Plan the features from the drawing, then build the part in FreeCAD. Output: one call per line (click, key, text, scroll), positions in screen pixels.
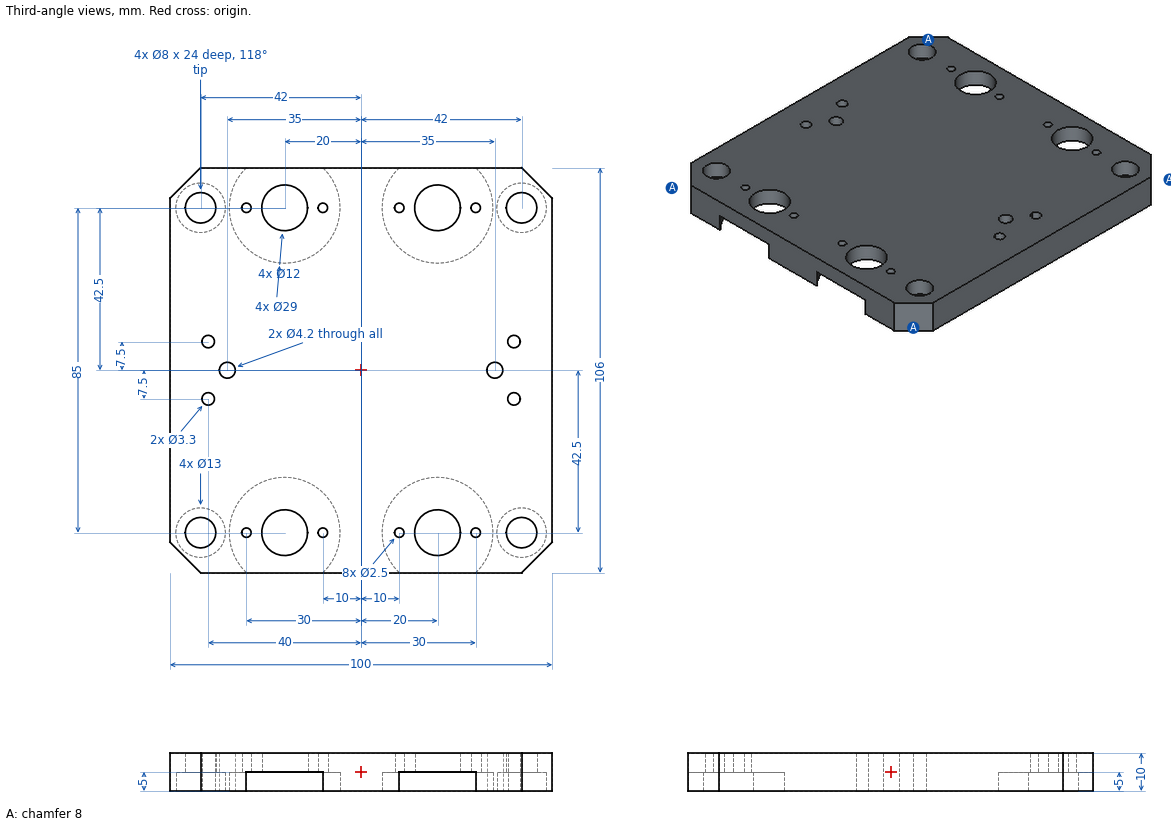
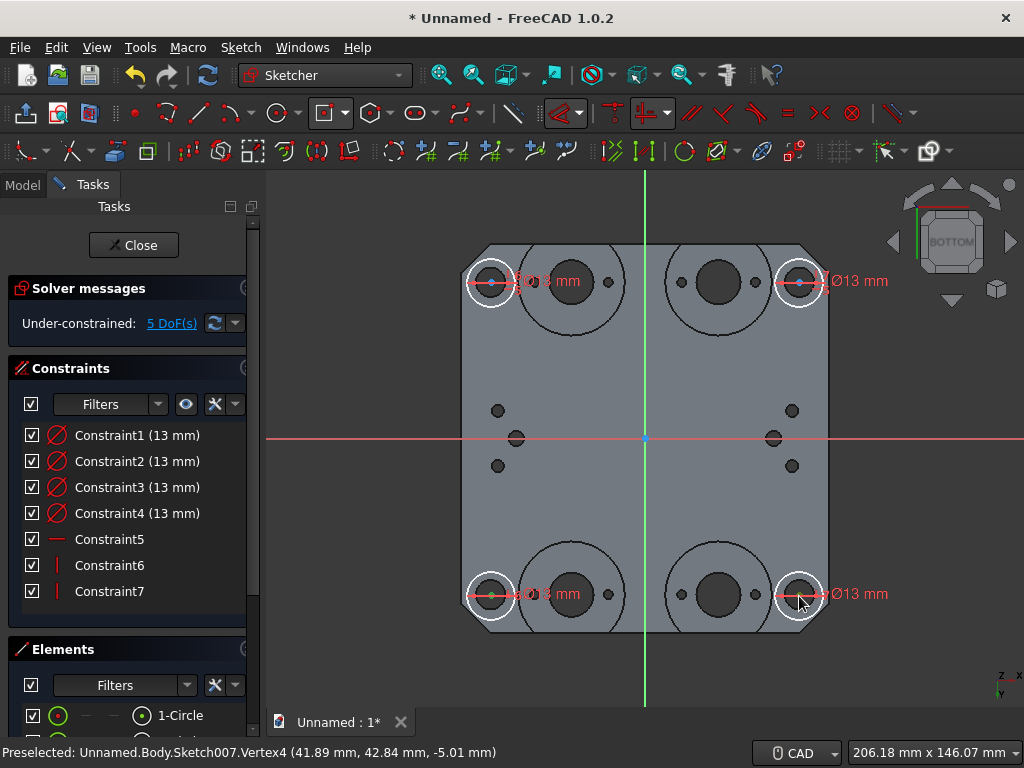
key(h)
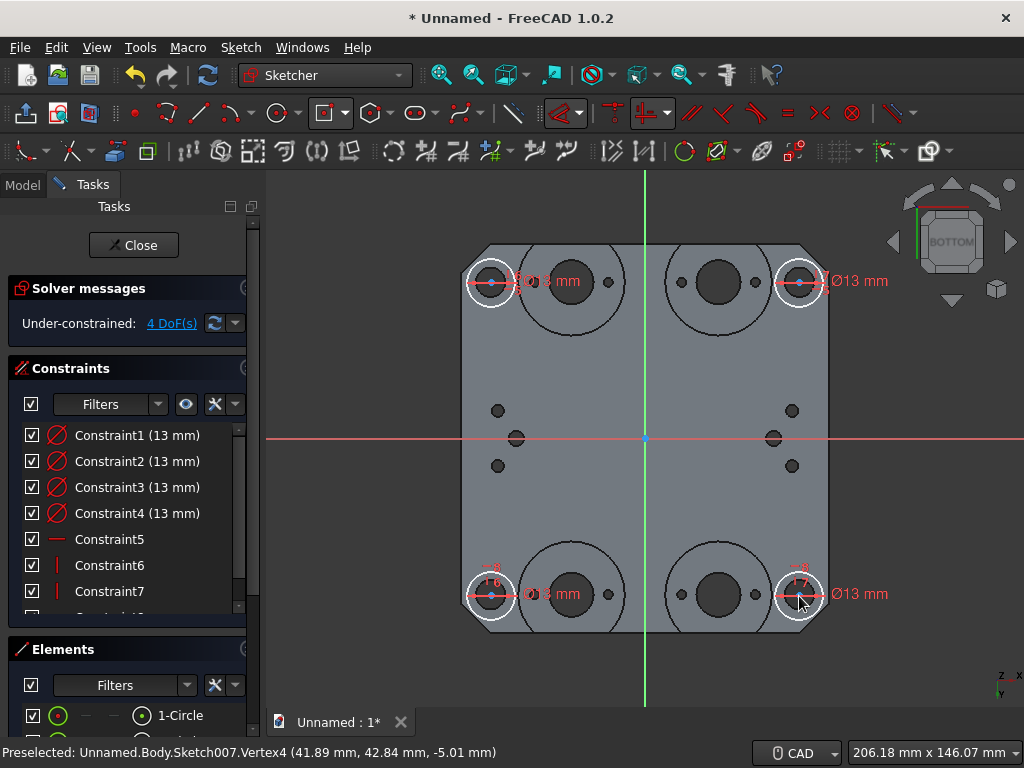
click(491, 283)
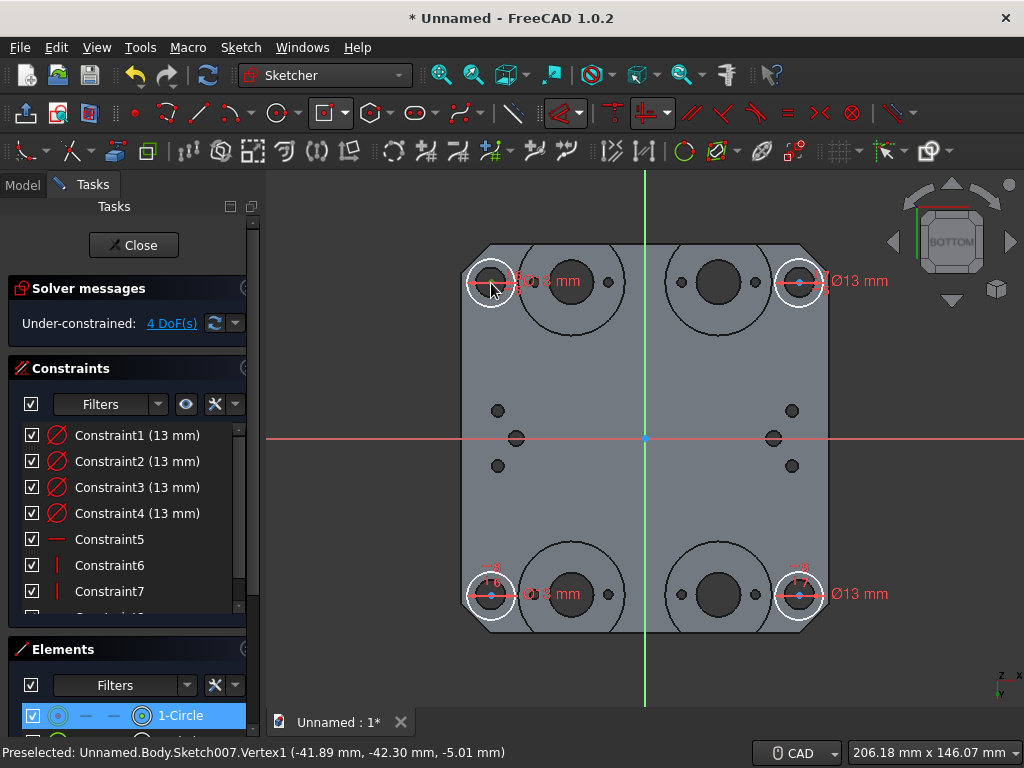
click(582, 114)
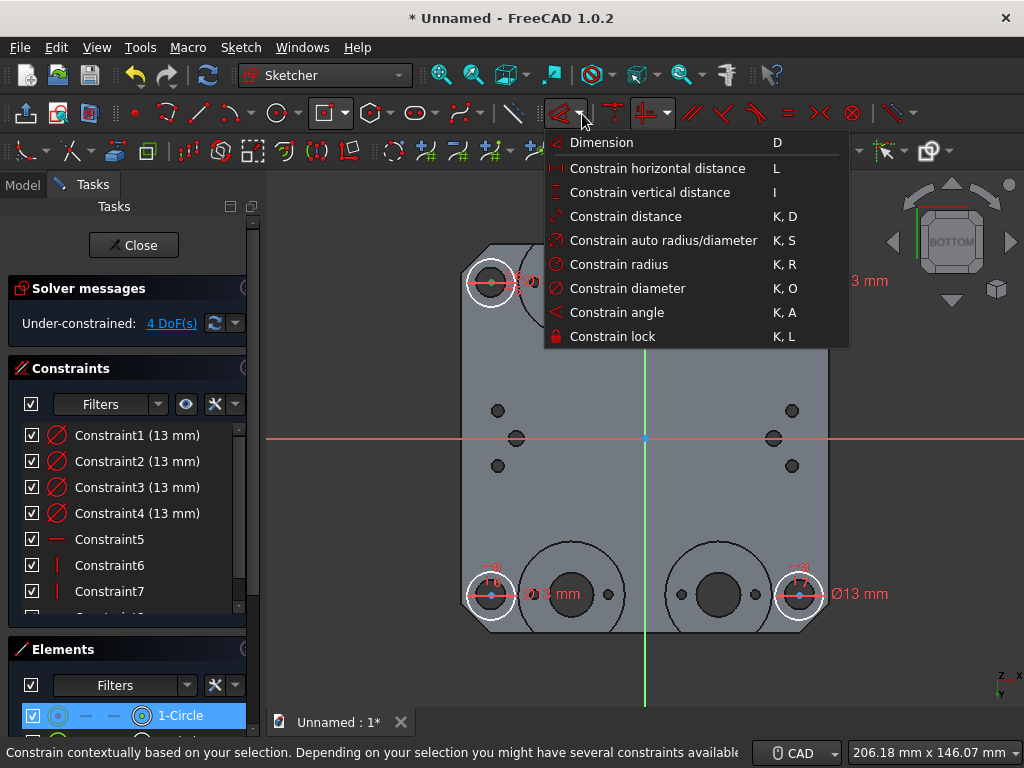
click(697, 168)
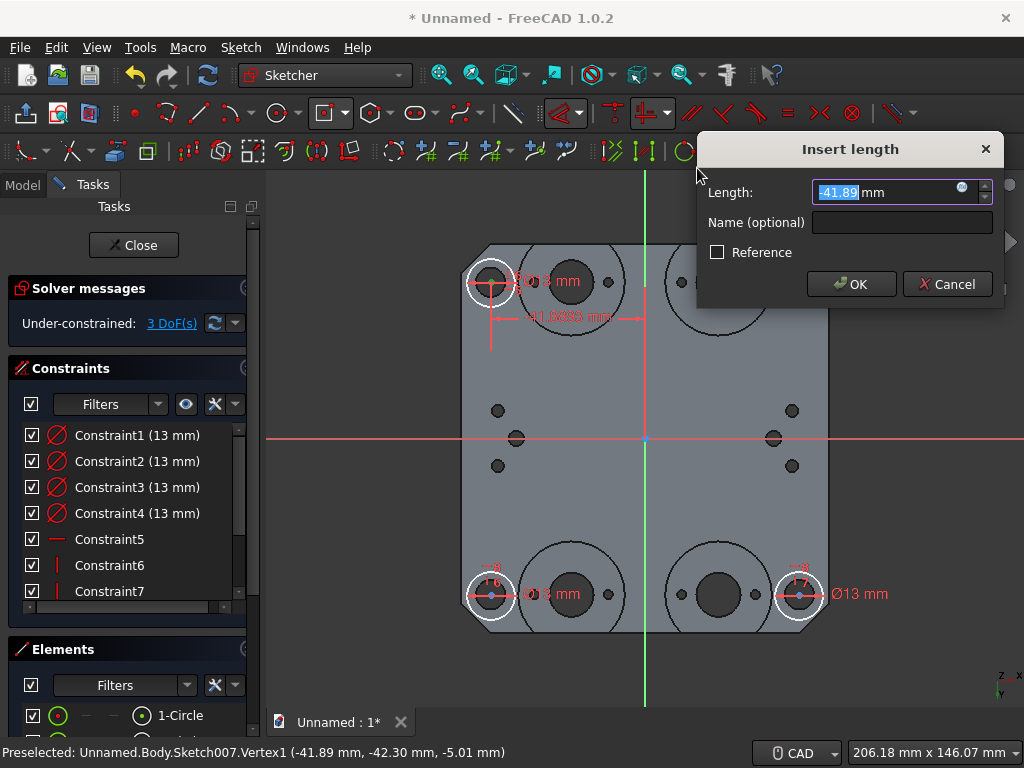
text(-42)
key(Return)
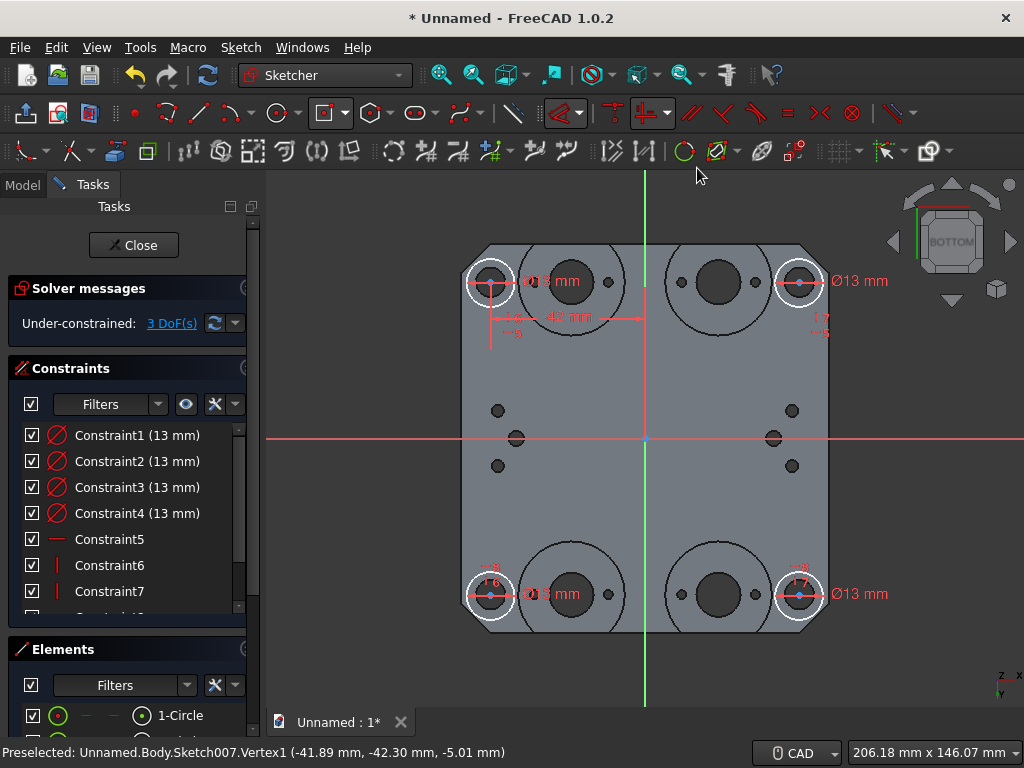
click(799, 283)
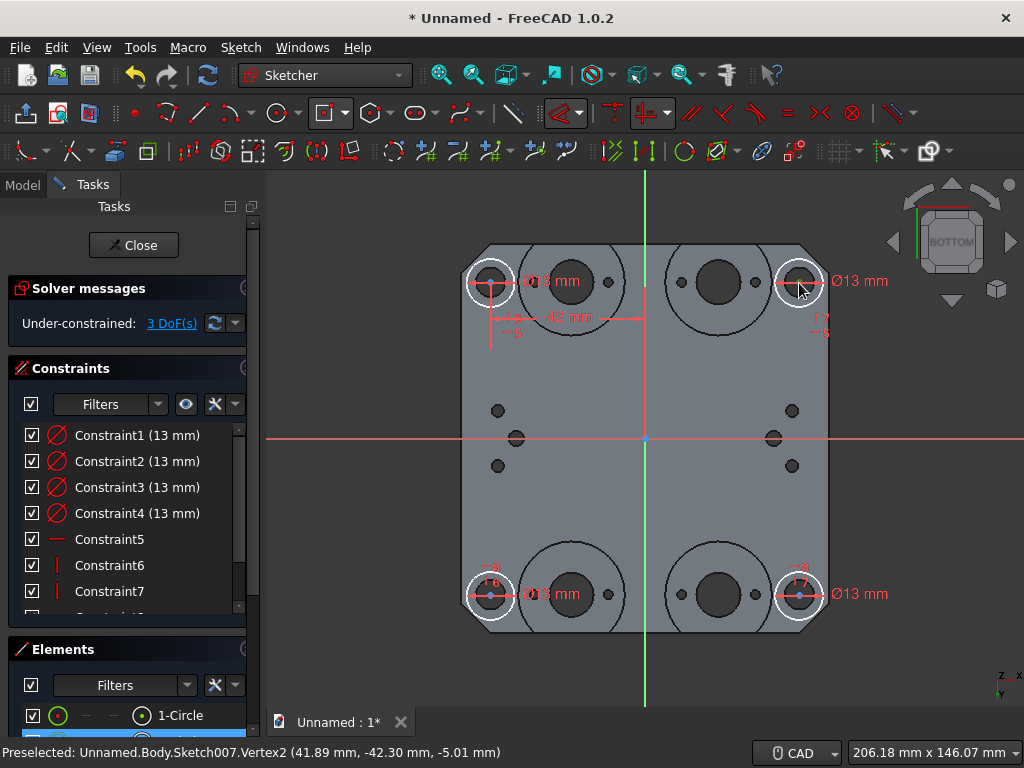
click(582, 114)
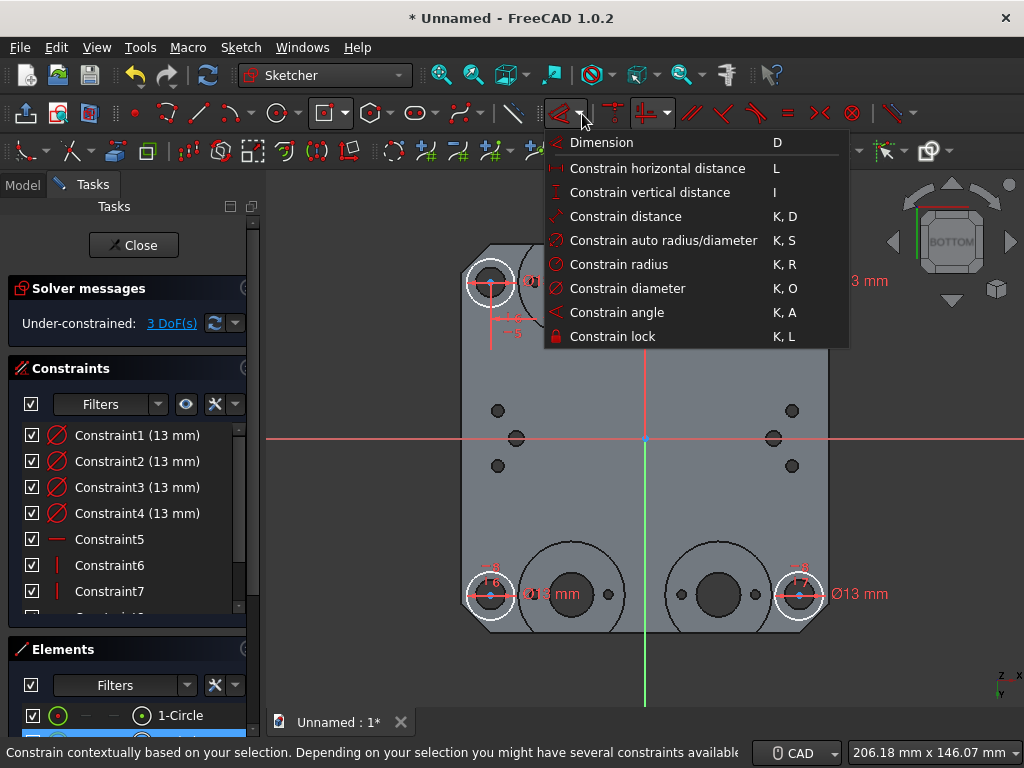
click(697, 168)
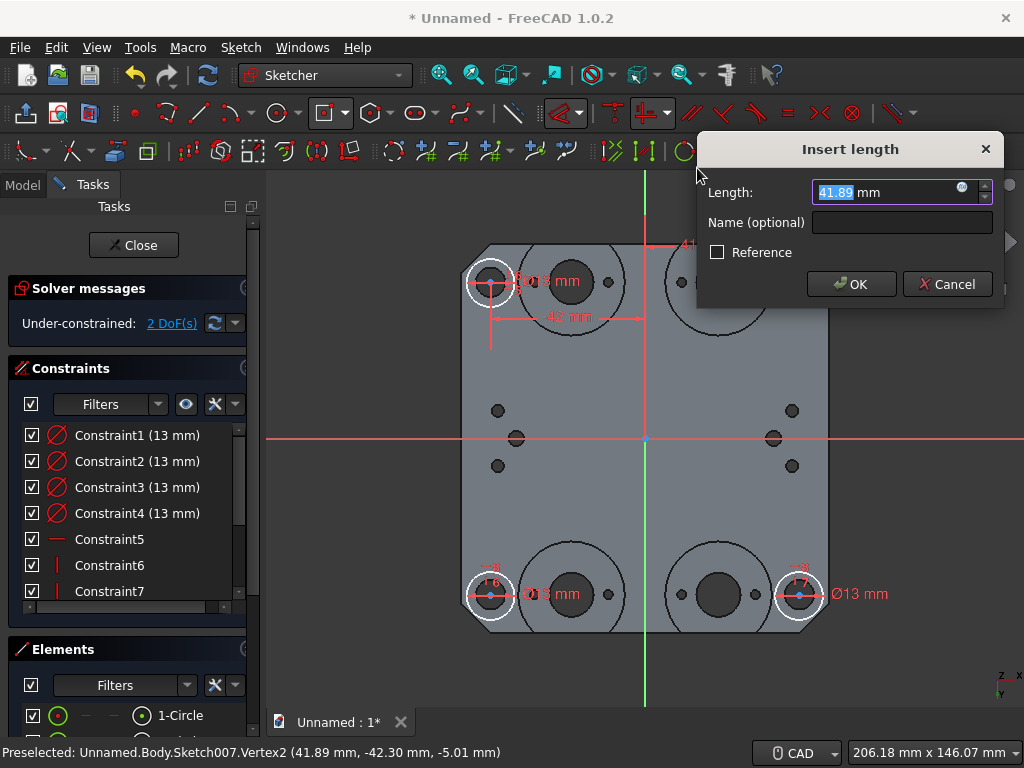
text(42)
key(Return)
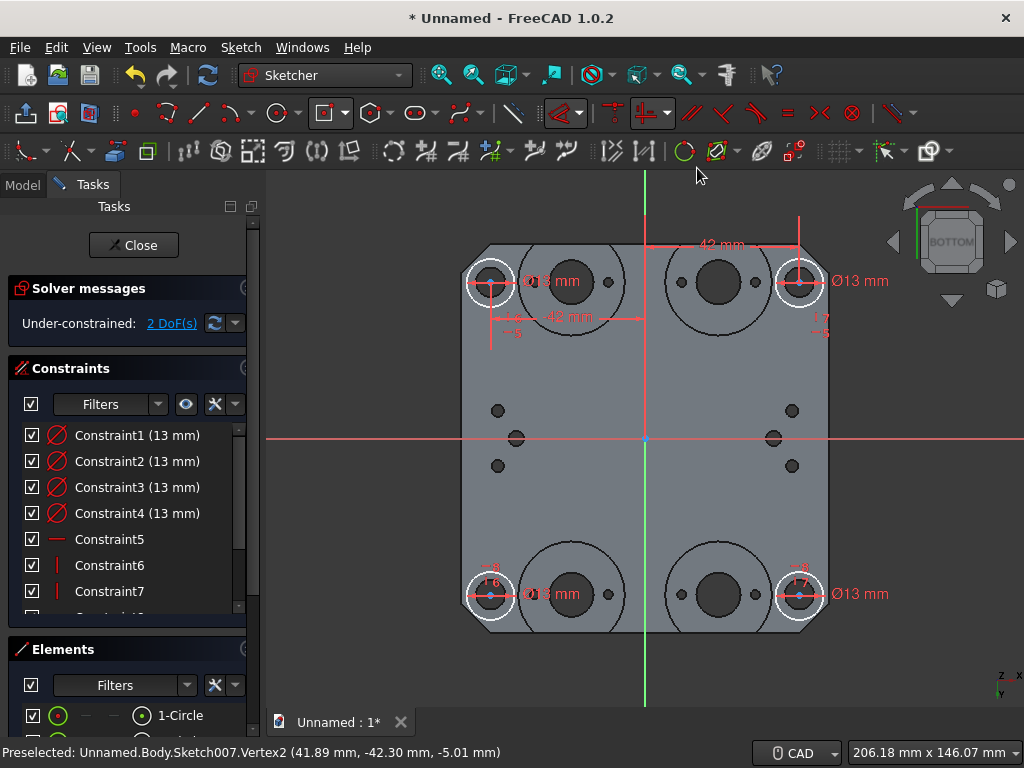
click(491, 283)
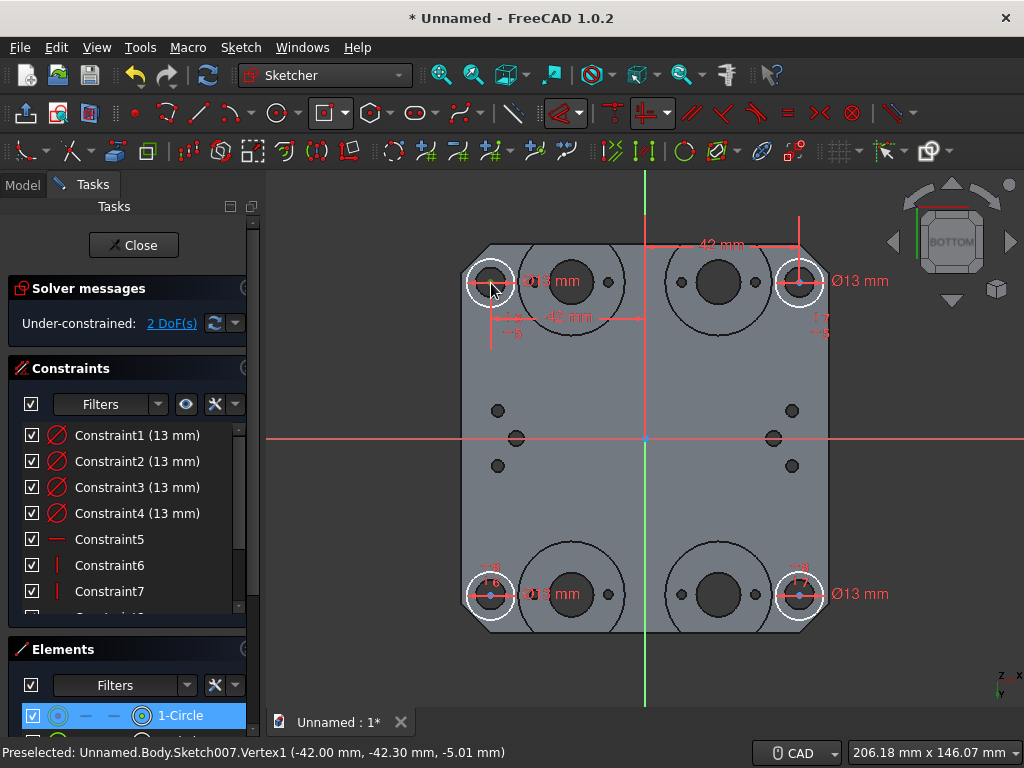
click(491, 596)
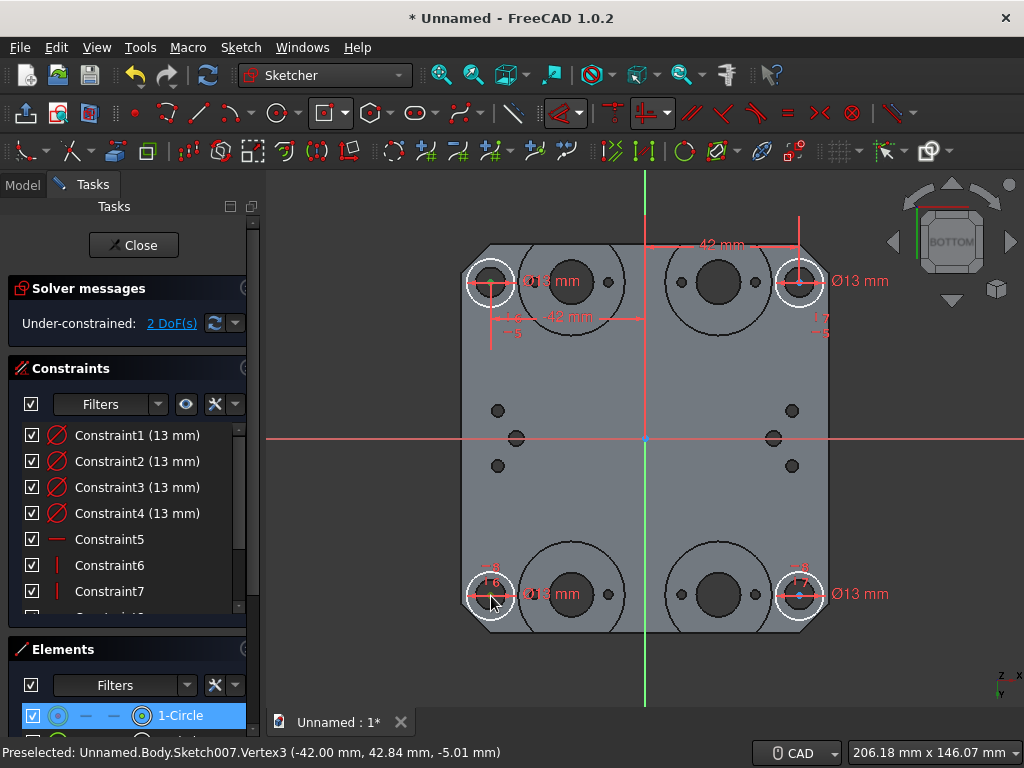
key(i)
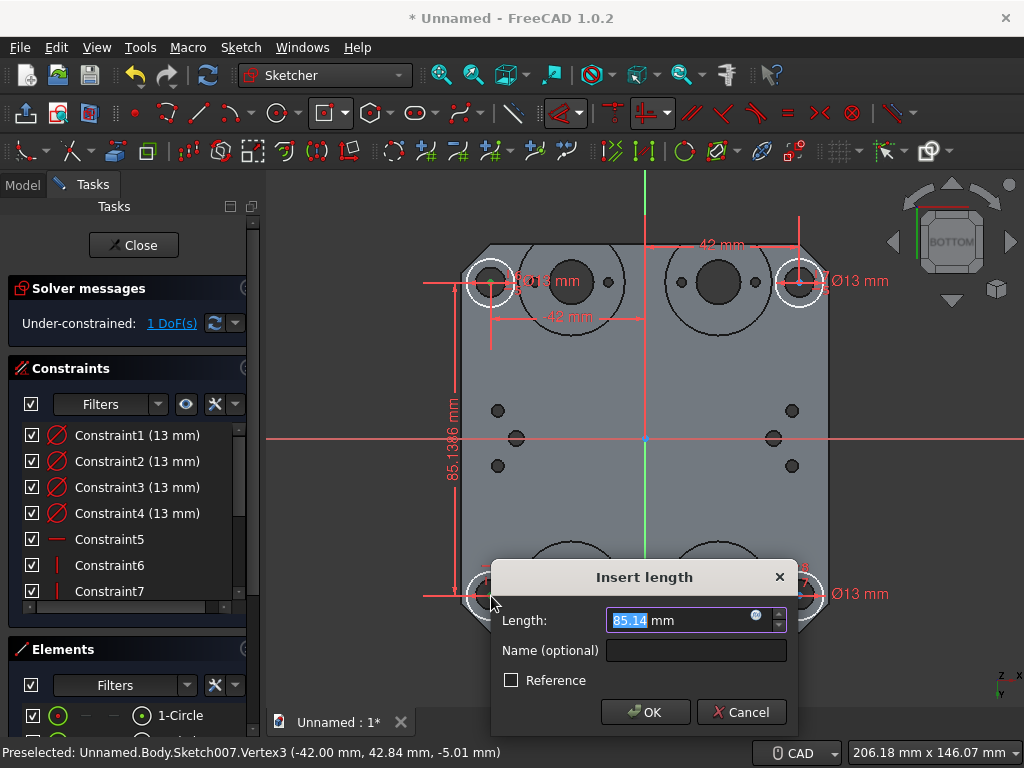
text(85)
key(Return)